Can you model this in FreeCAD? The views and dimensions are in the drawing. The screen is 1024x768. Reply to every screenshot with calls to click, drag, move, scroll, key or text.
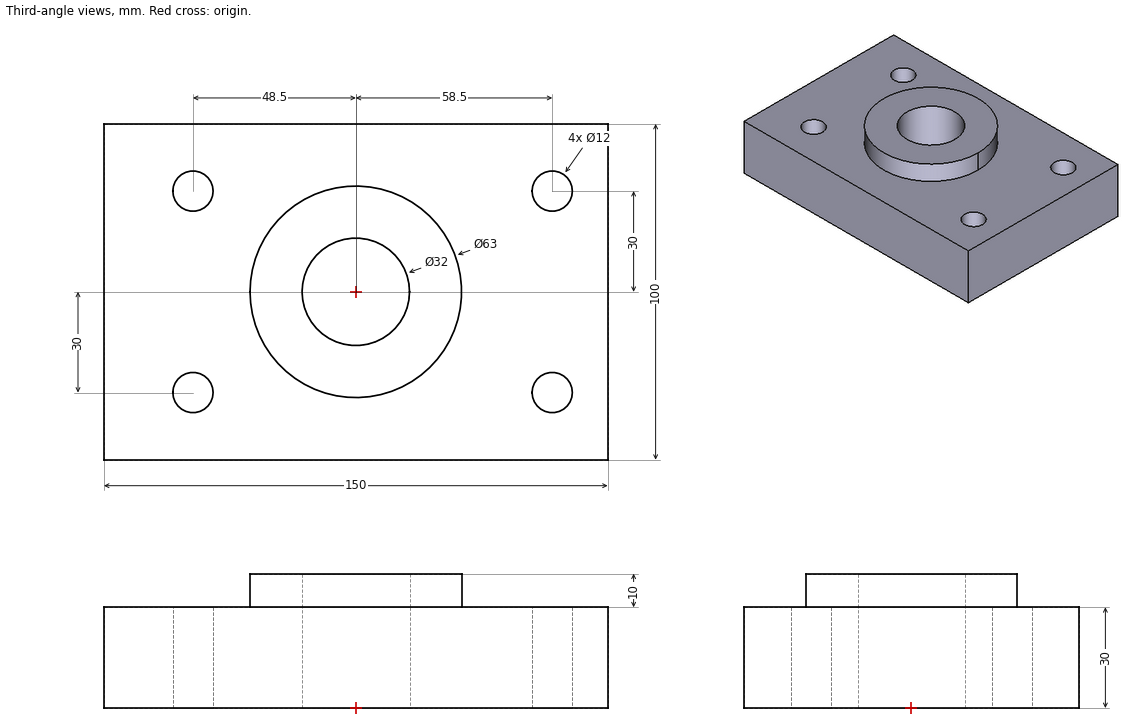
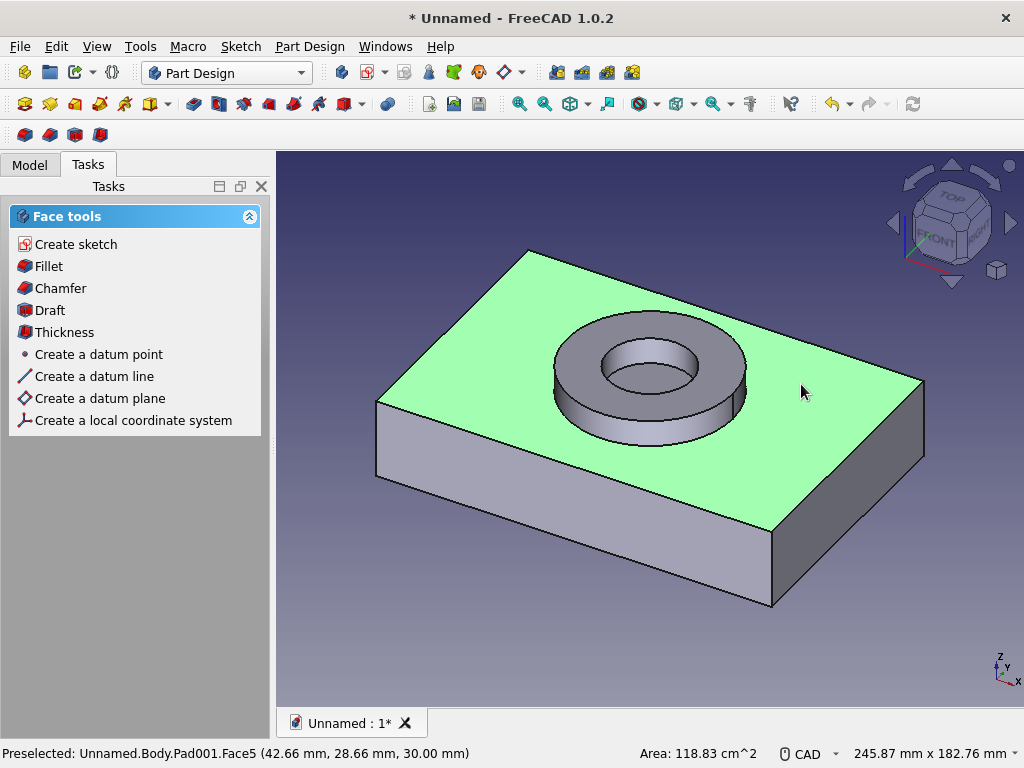
click(366, 72)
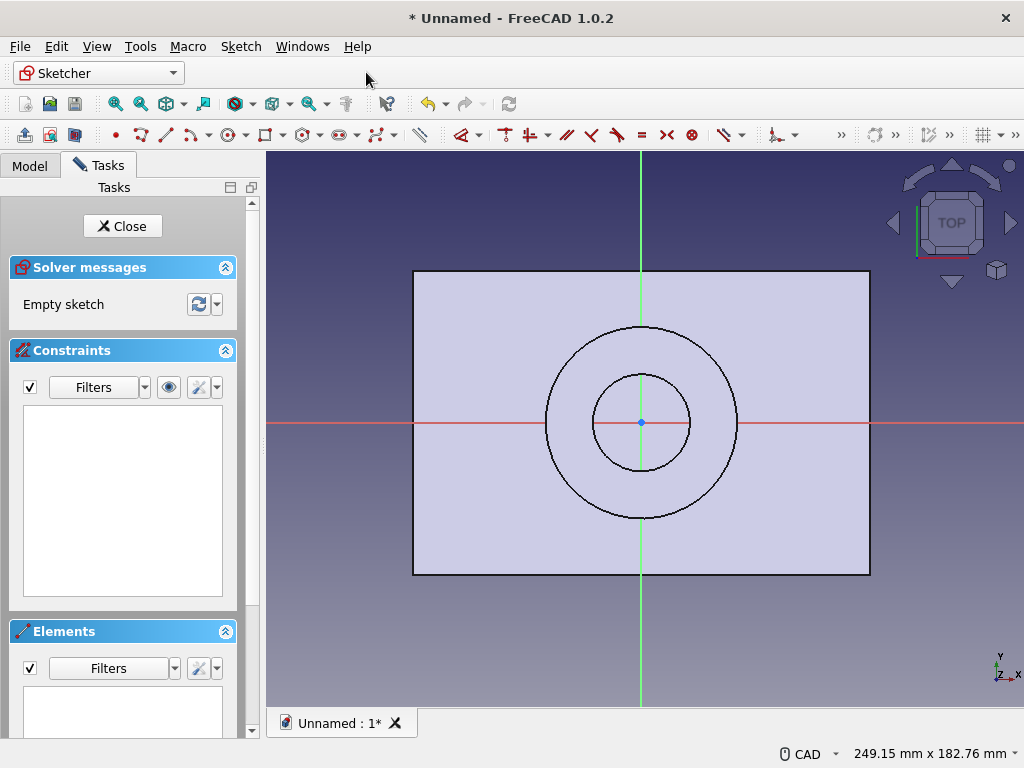
key(q)
key(s)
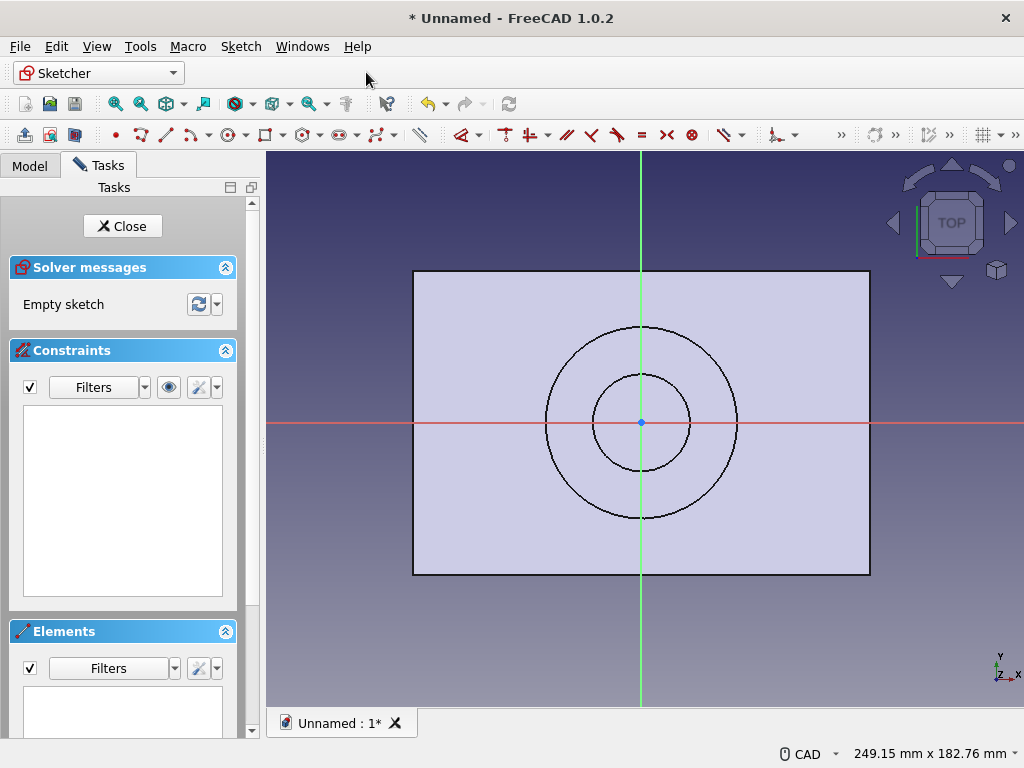
scroll(669, 420, up, 6)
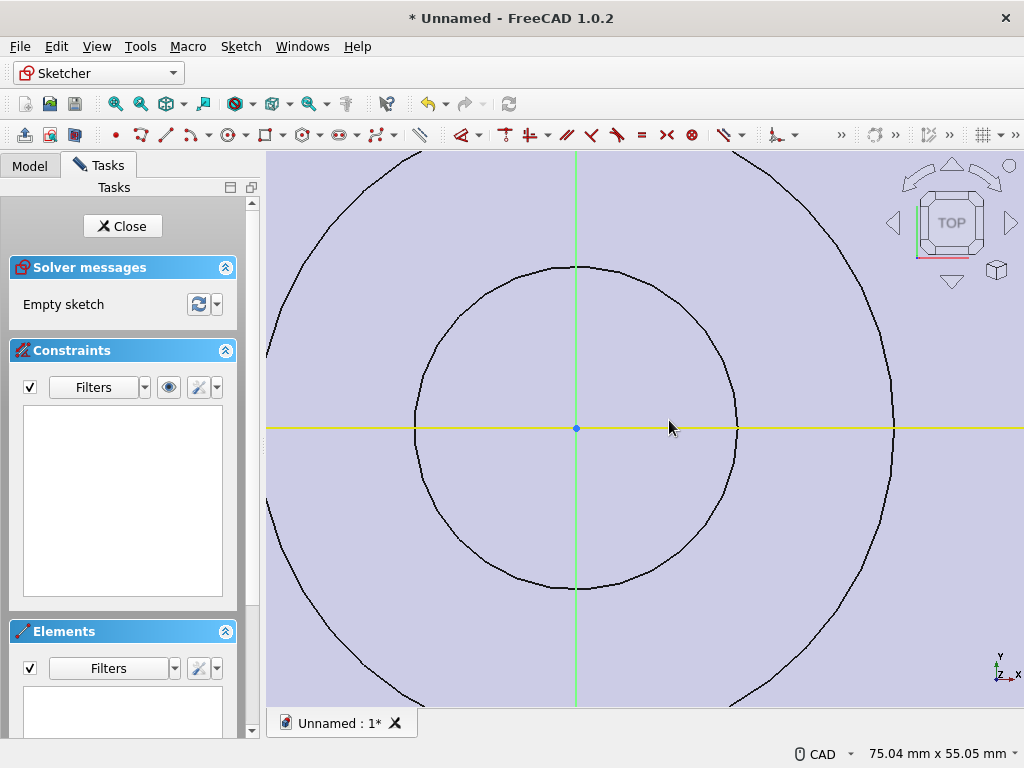
click(228, 136)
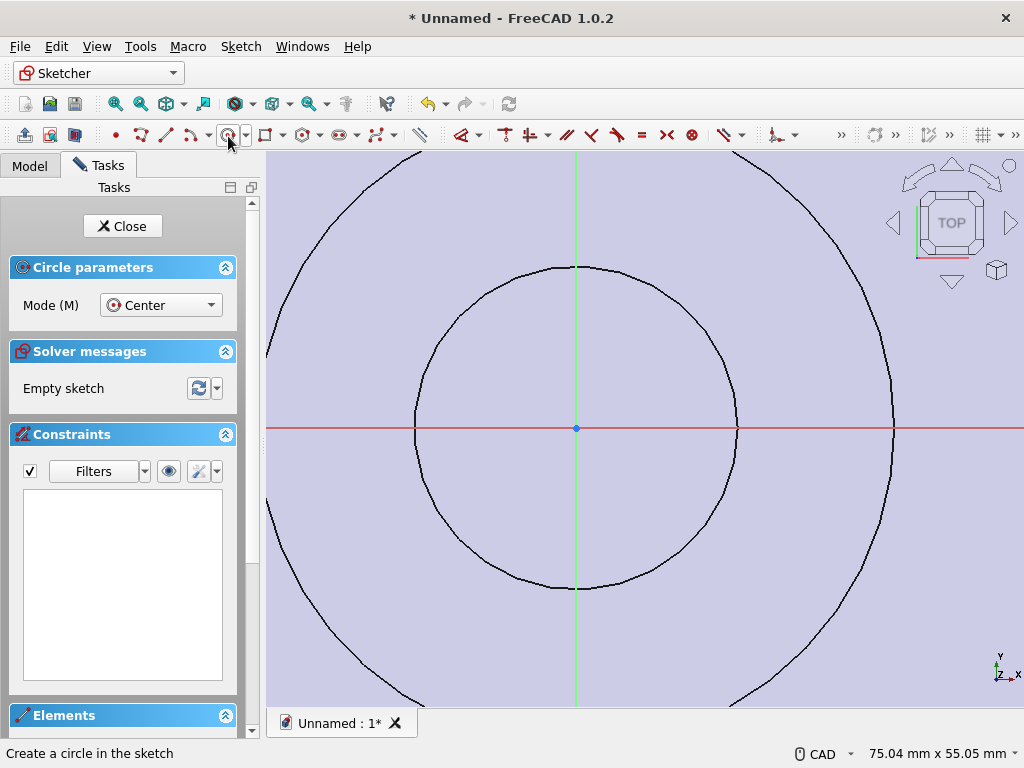
click(576, 428)
move(690, 314)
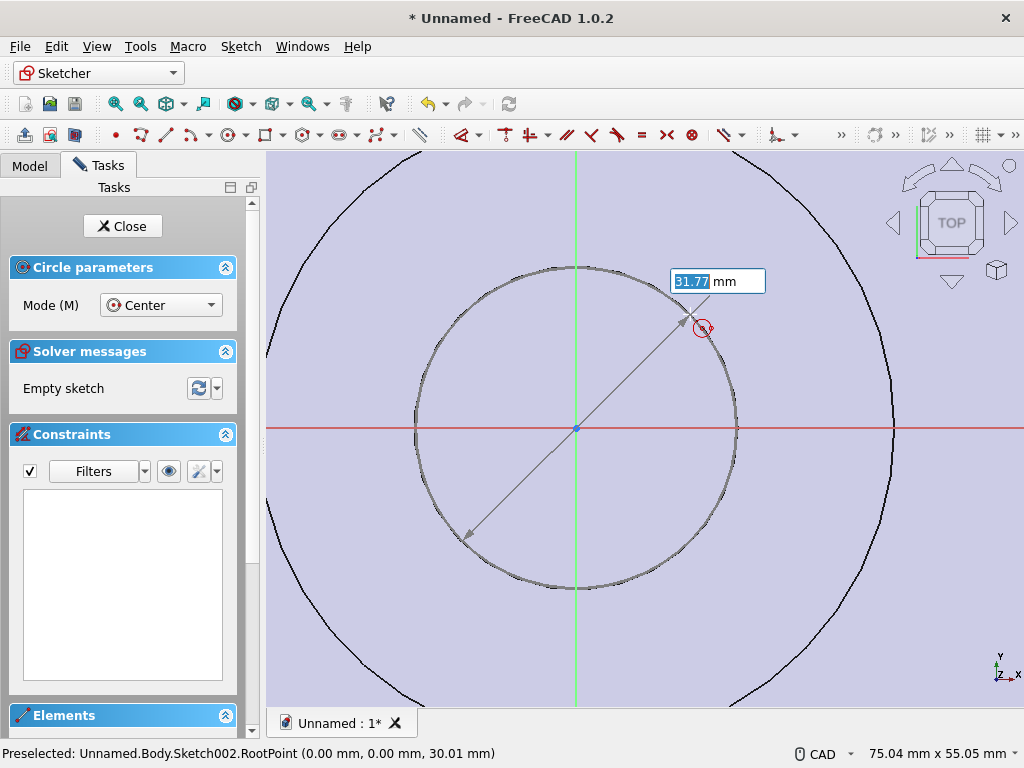
text(32)
key(Return)
key(Escape)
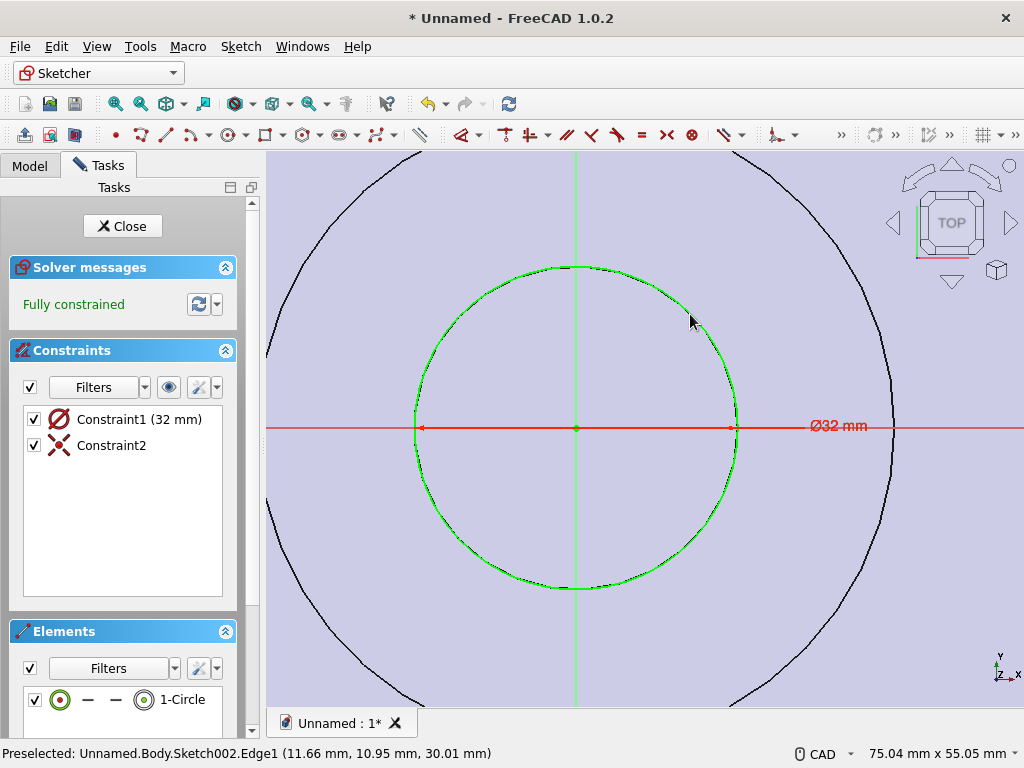
click(123, 226)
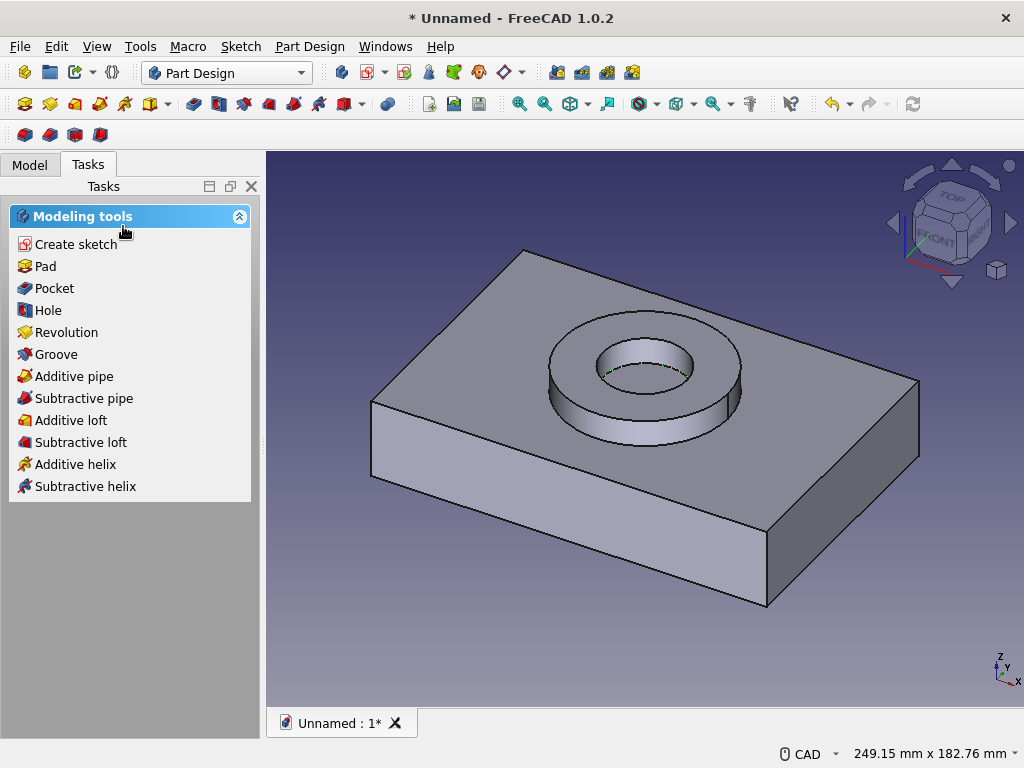
click(194, 104)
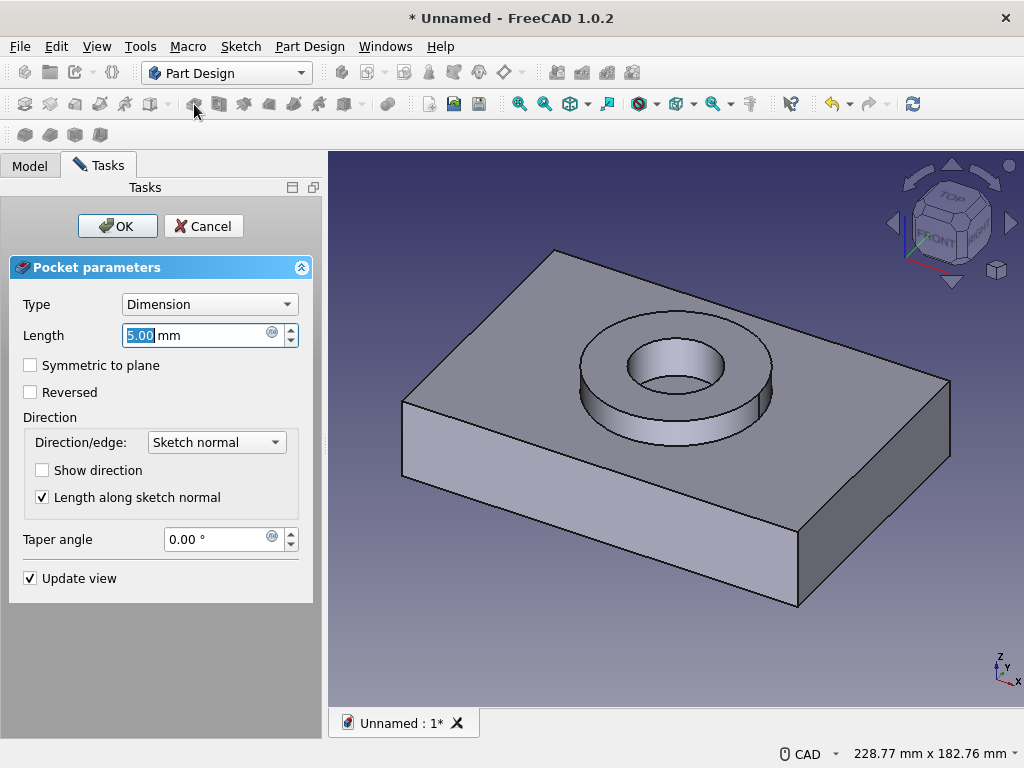
click(210, 304)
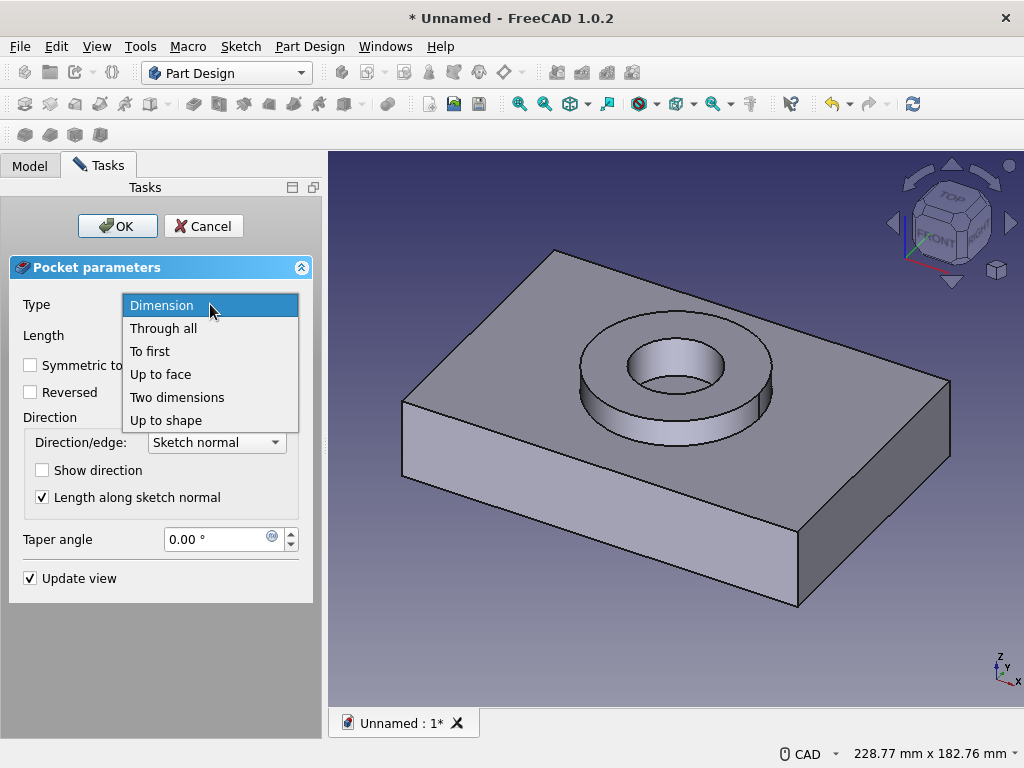
click(208, 328)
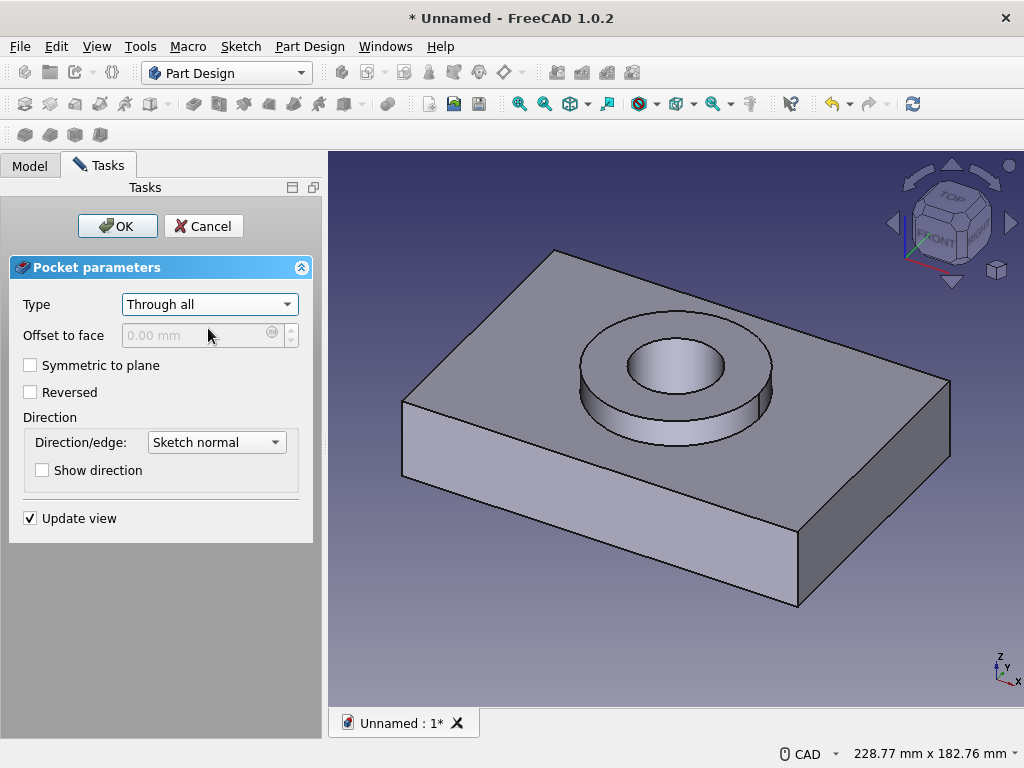
click(118, 226)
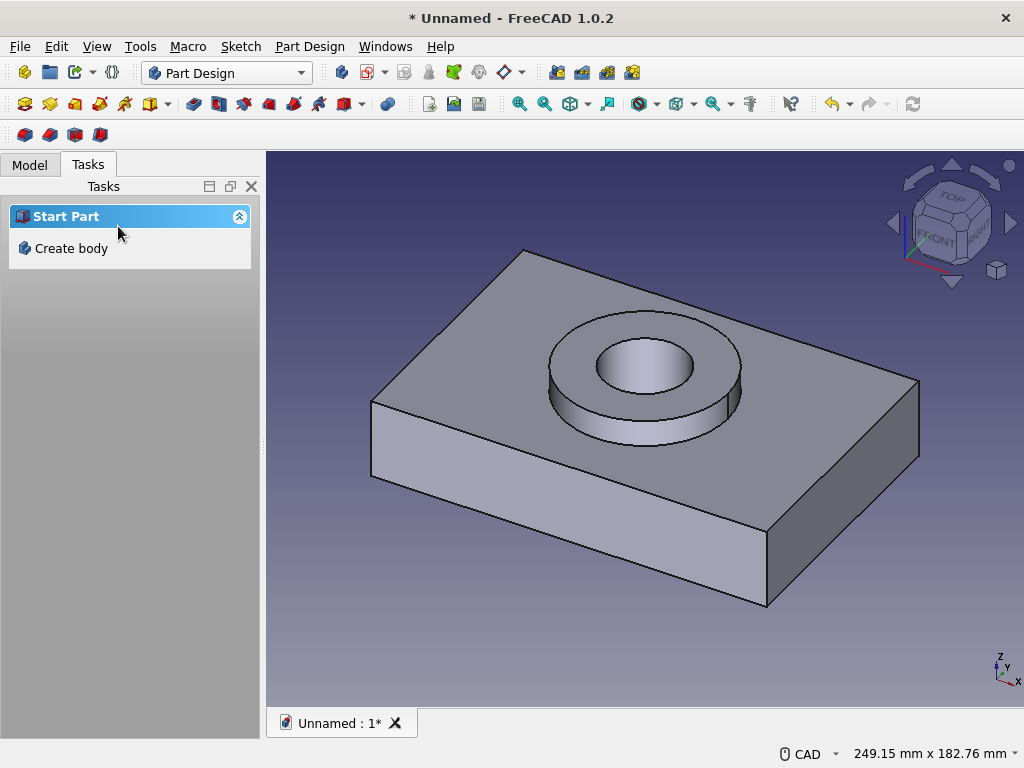
click(366, 72)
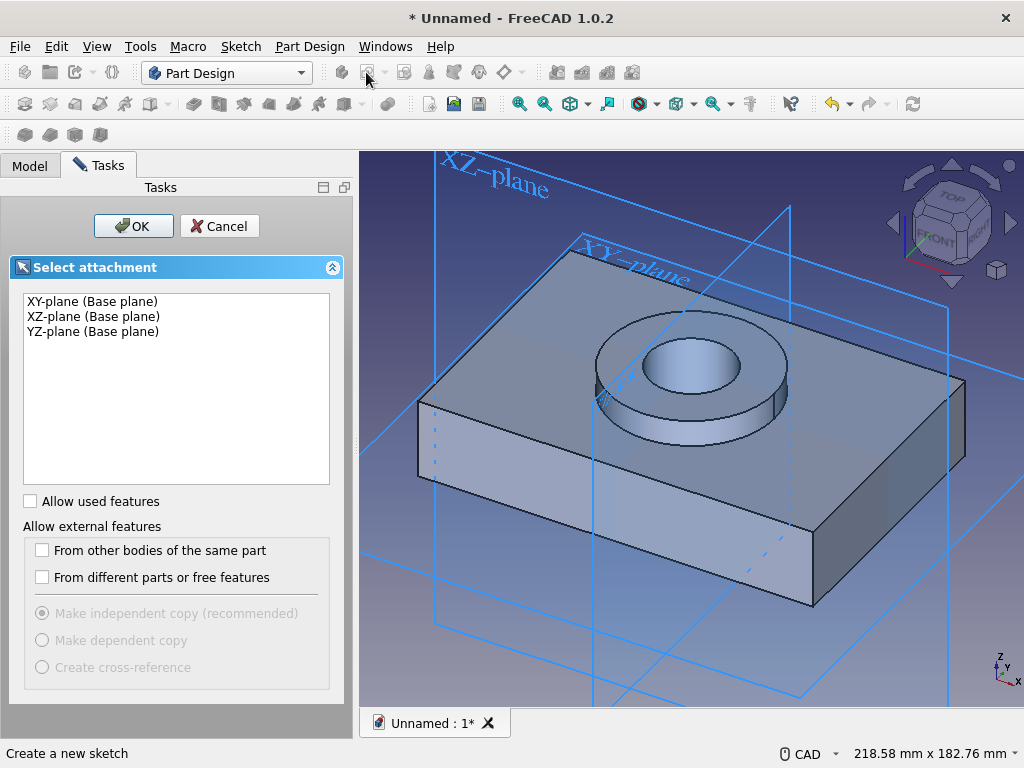
click(84, 302)